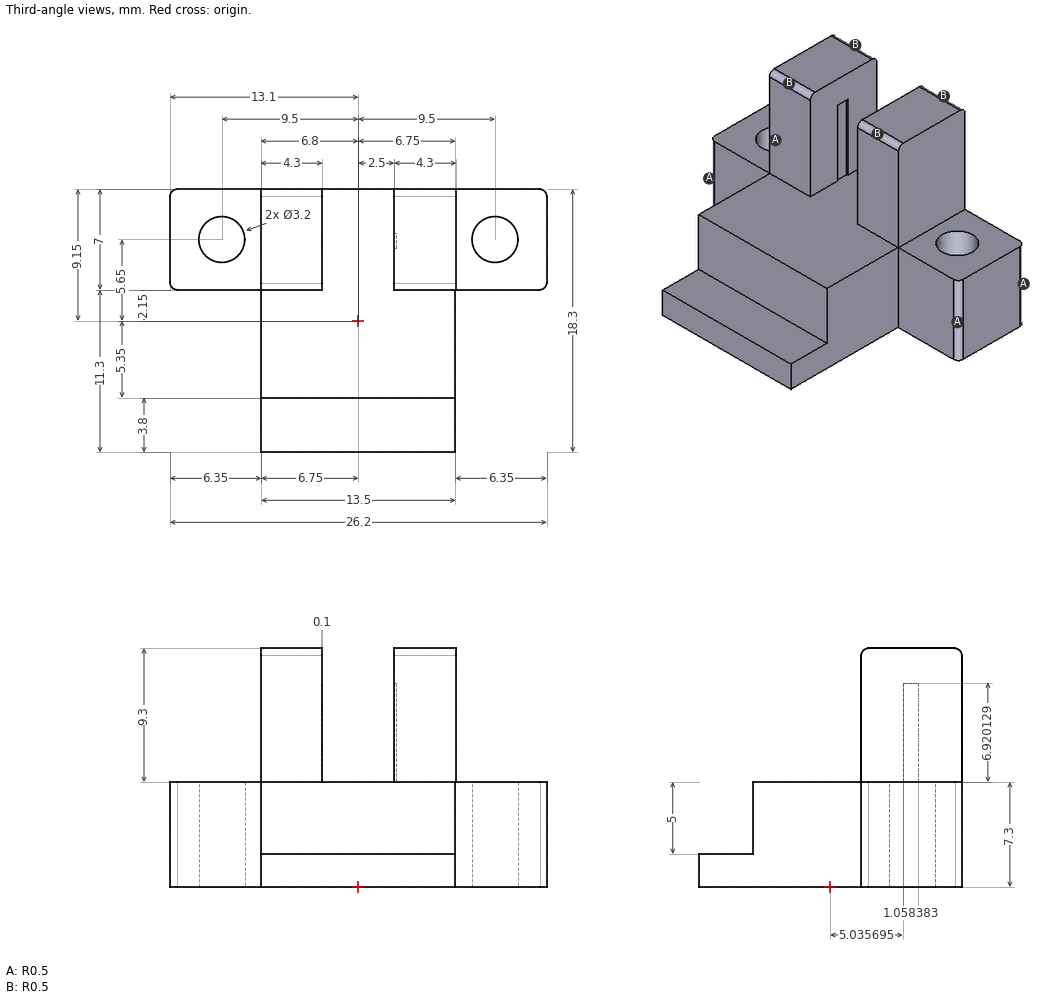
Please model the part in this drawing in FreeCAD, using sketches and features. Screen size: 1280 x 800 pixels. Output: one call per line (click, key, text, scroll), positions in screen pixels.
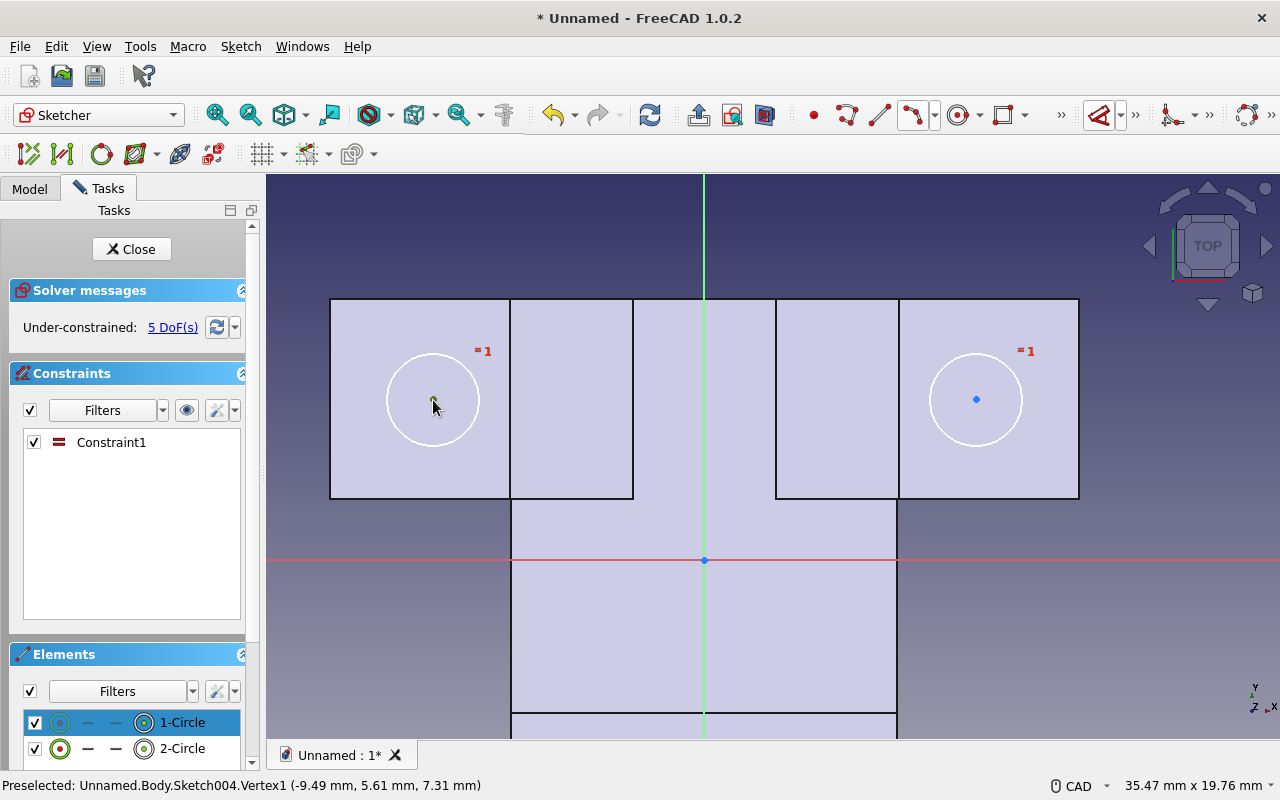
click(976, 400)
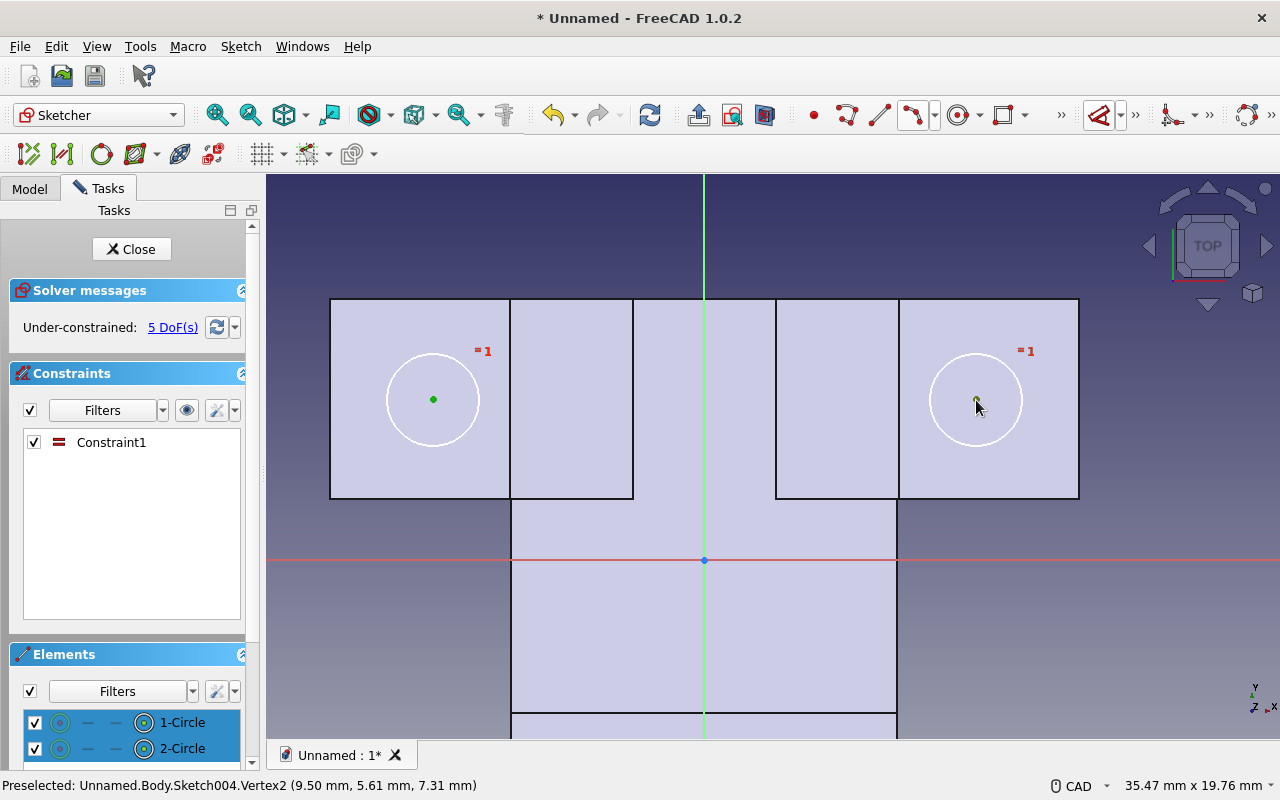
key(h)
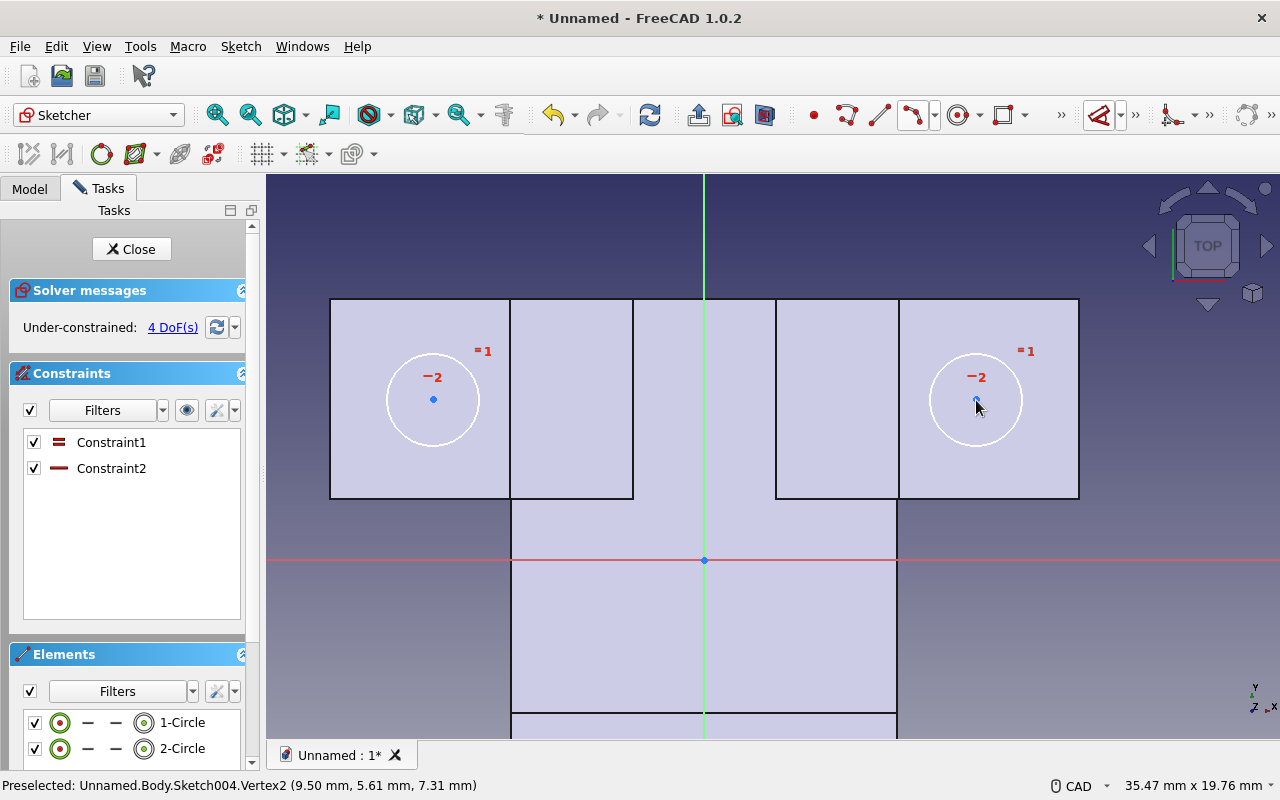
click(465, 367)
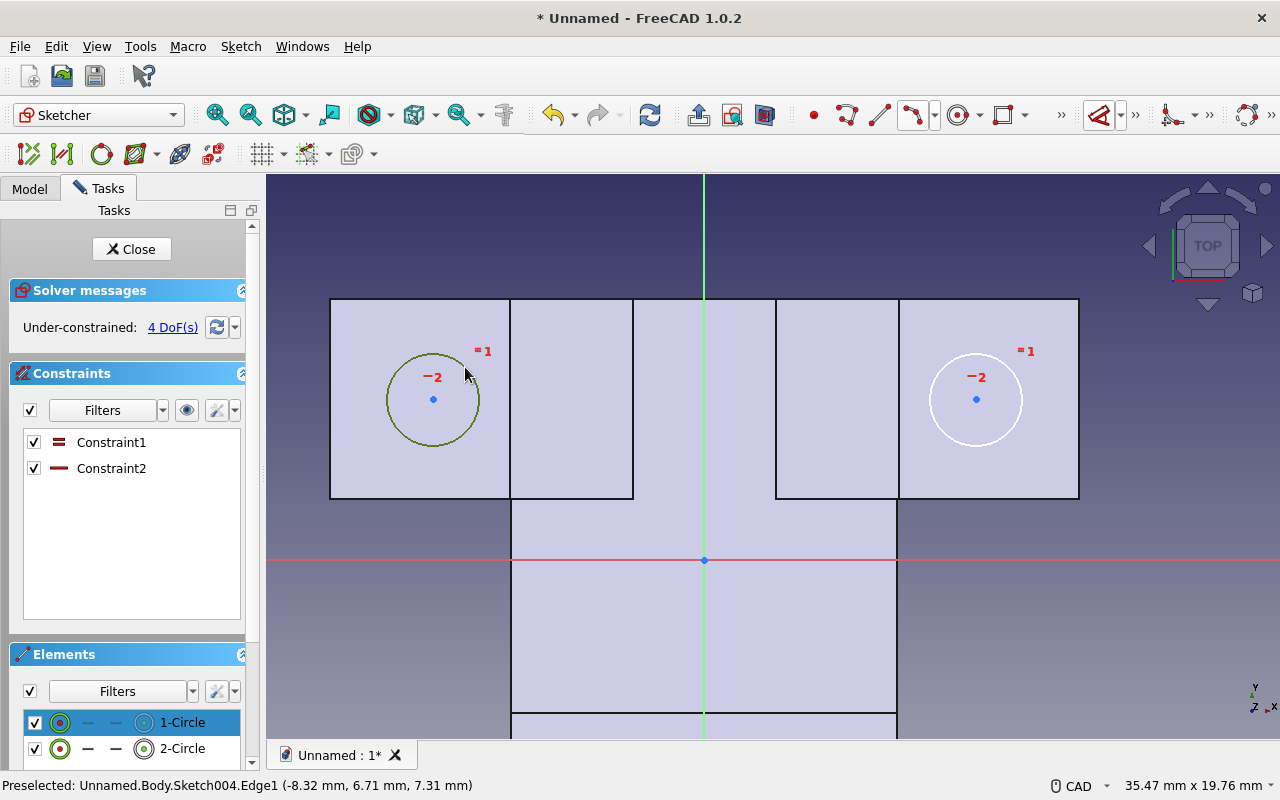
key(k)
key(o)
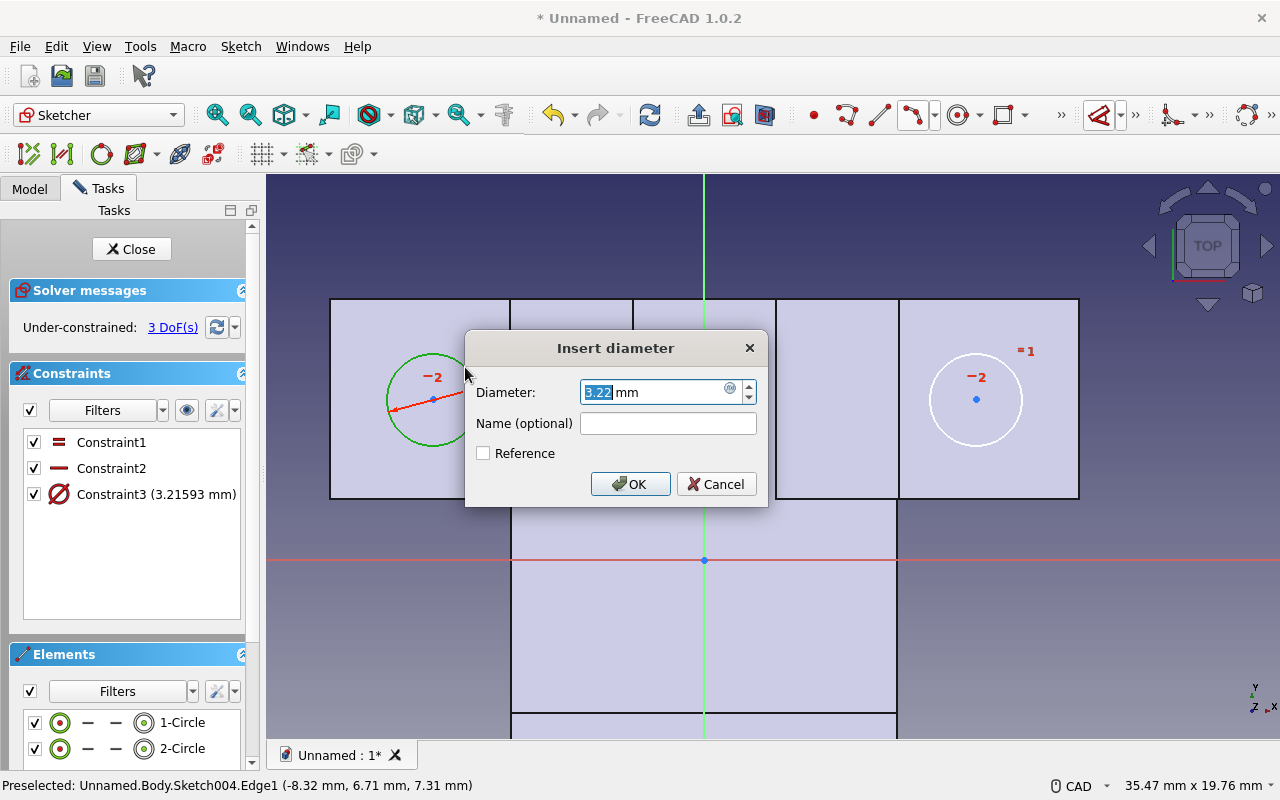
text(3.2)
key(Return)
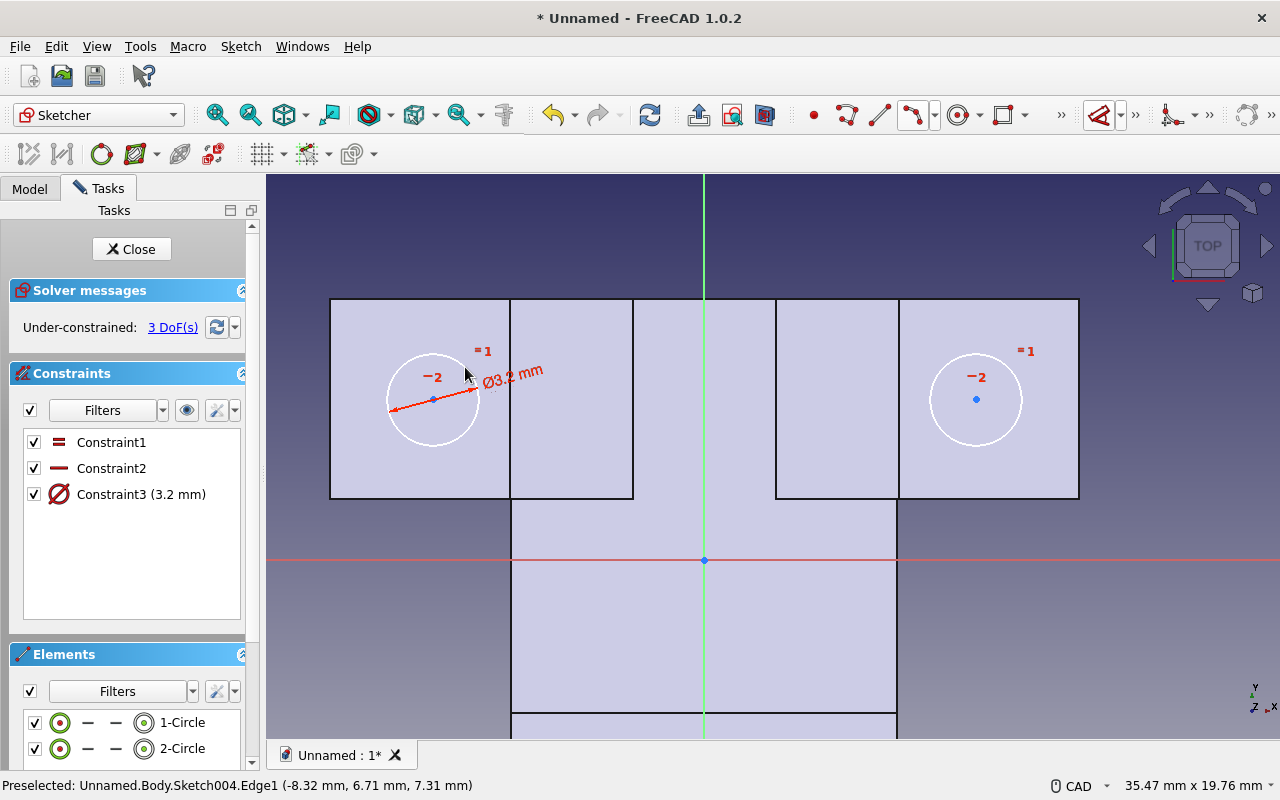
click(433, 400)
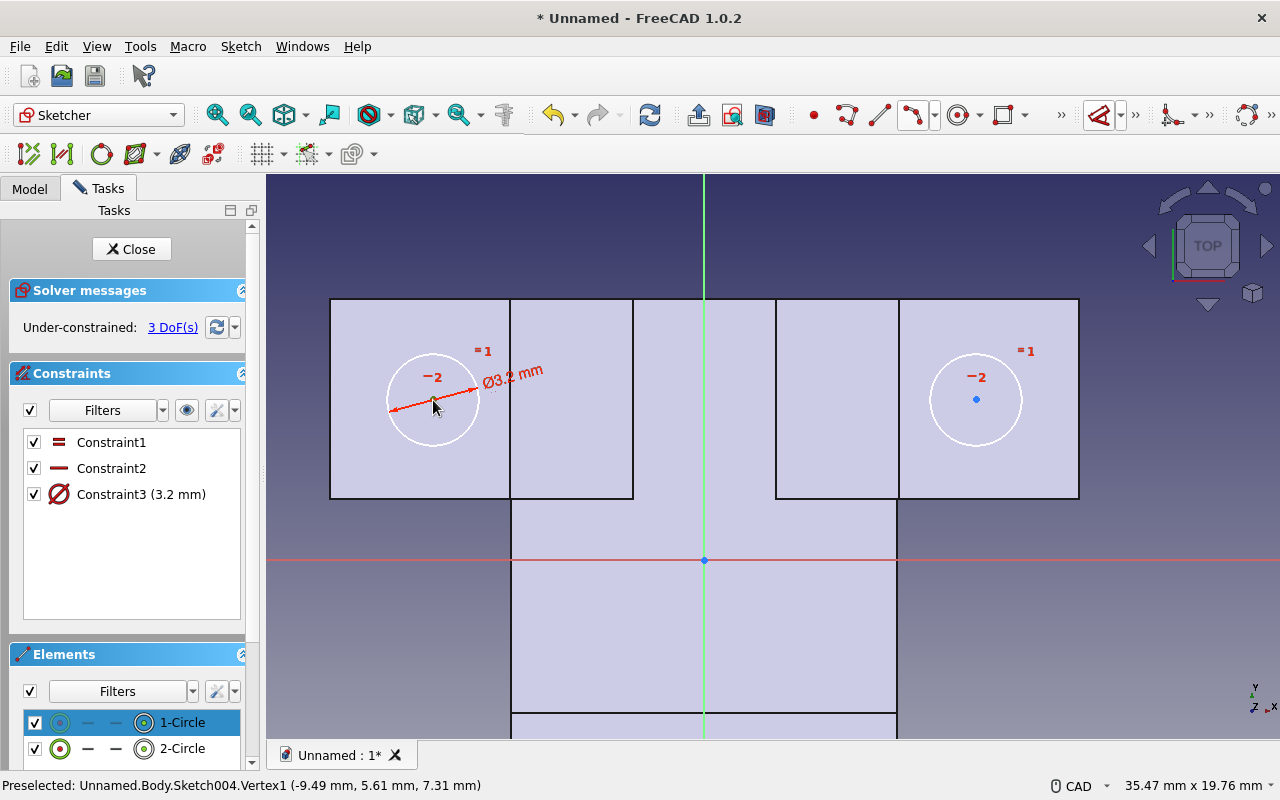
key(l)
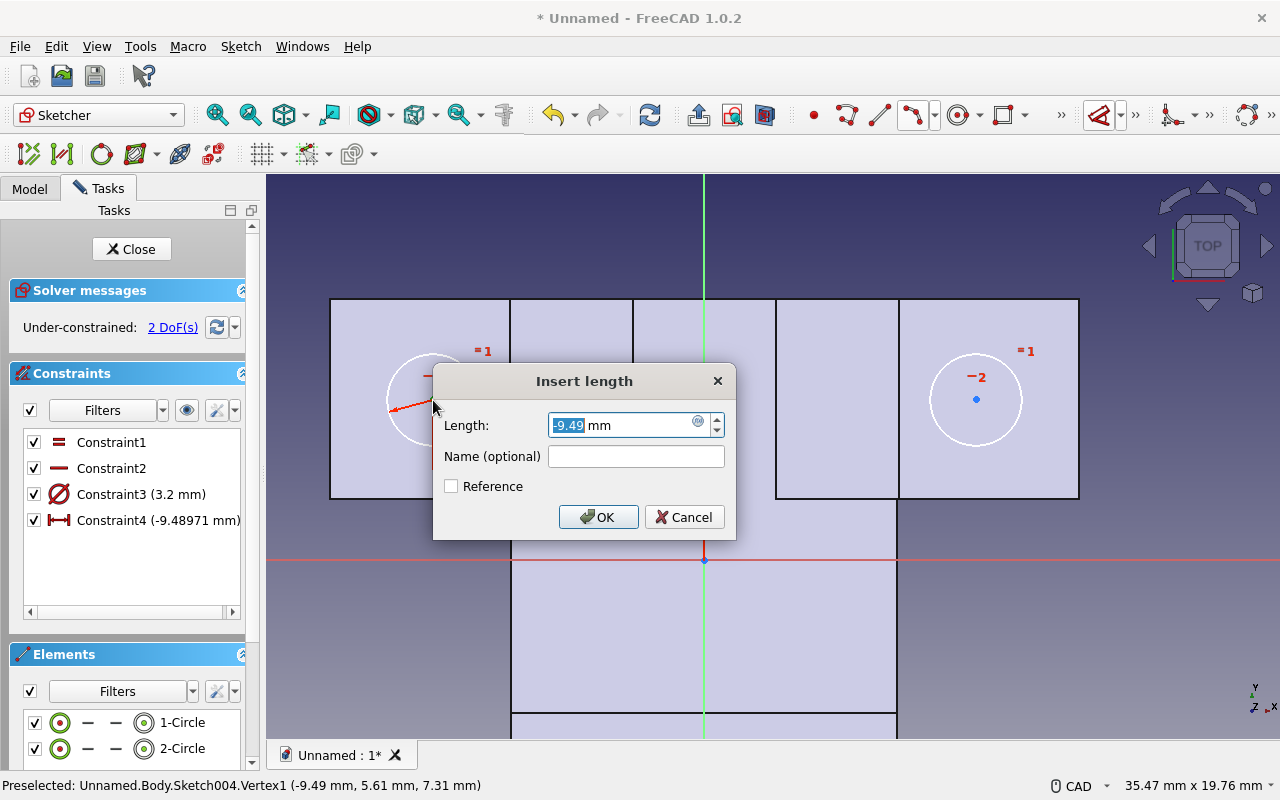
text(-9.5)
key(Return)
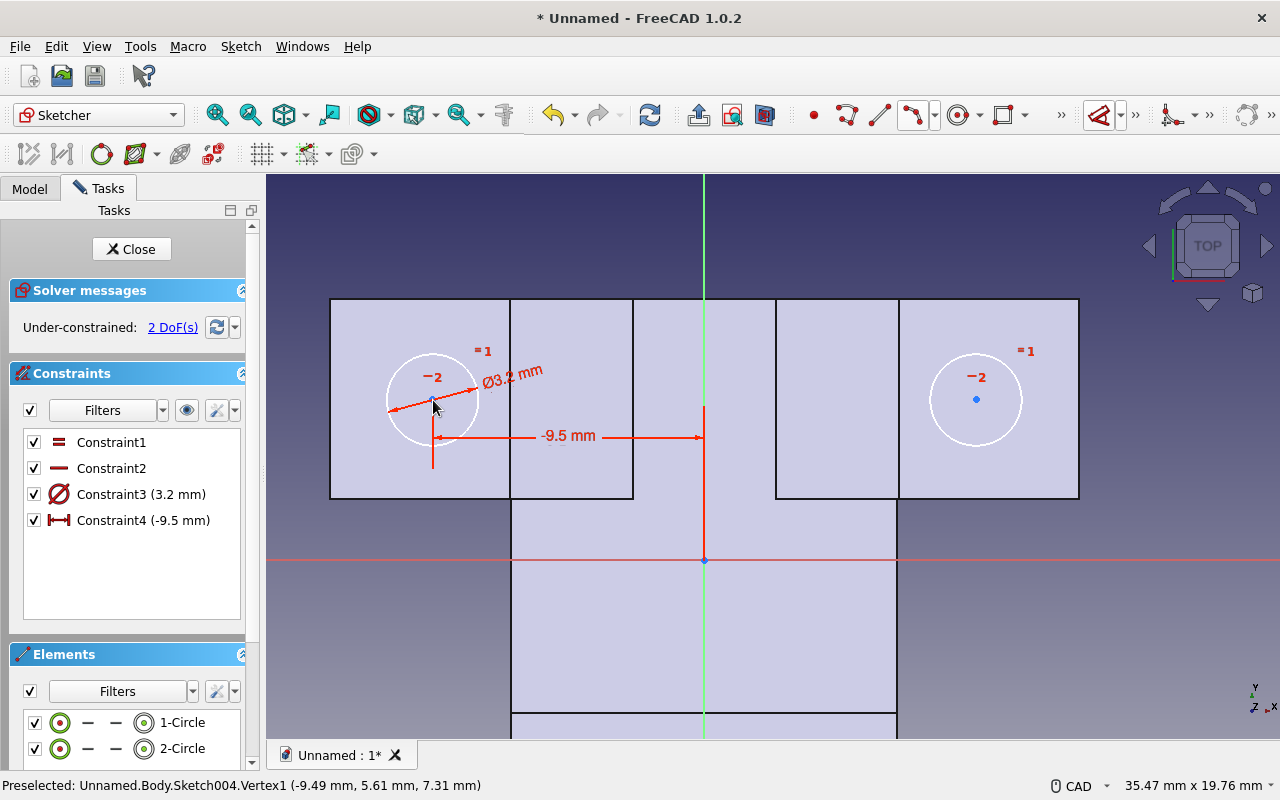
click(976, 400)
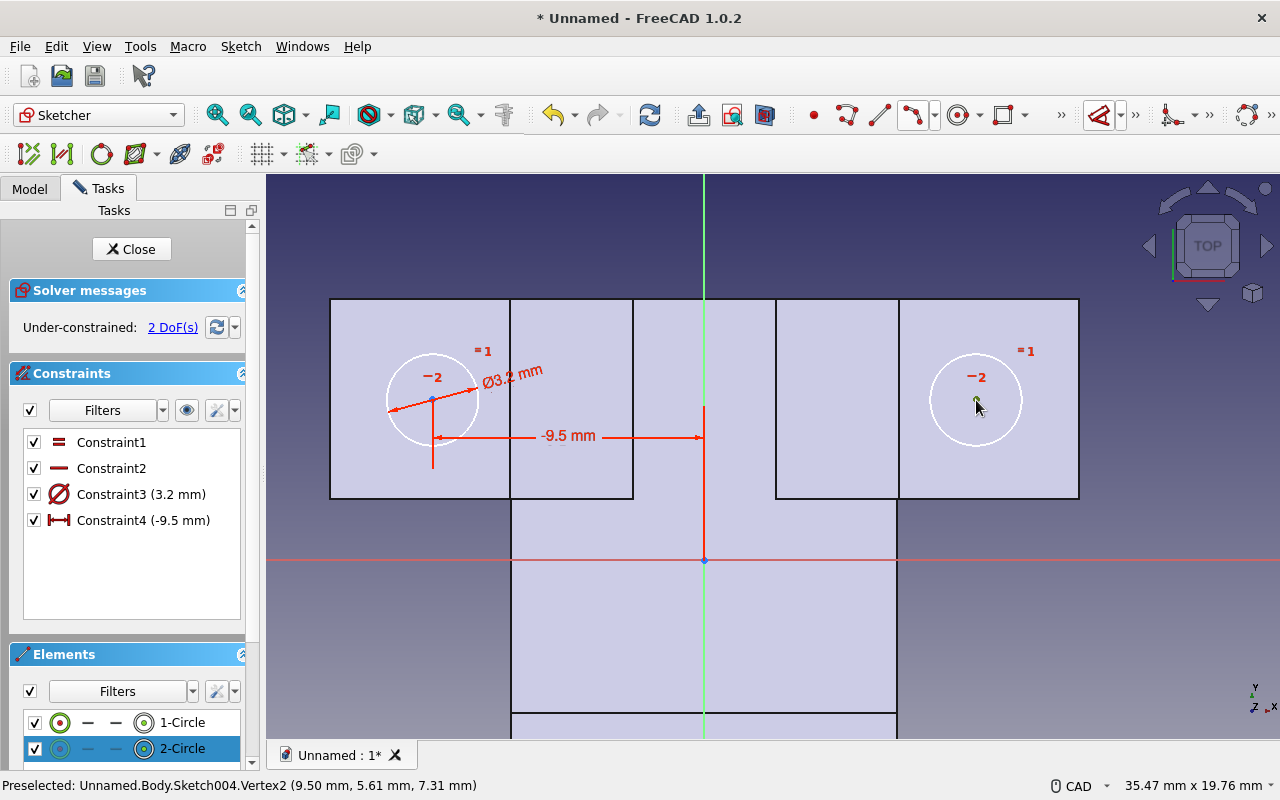
key(l)